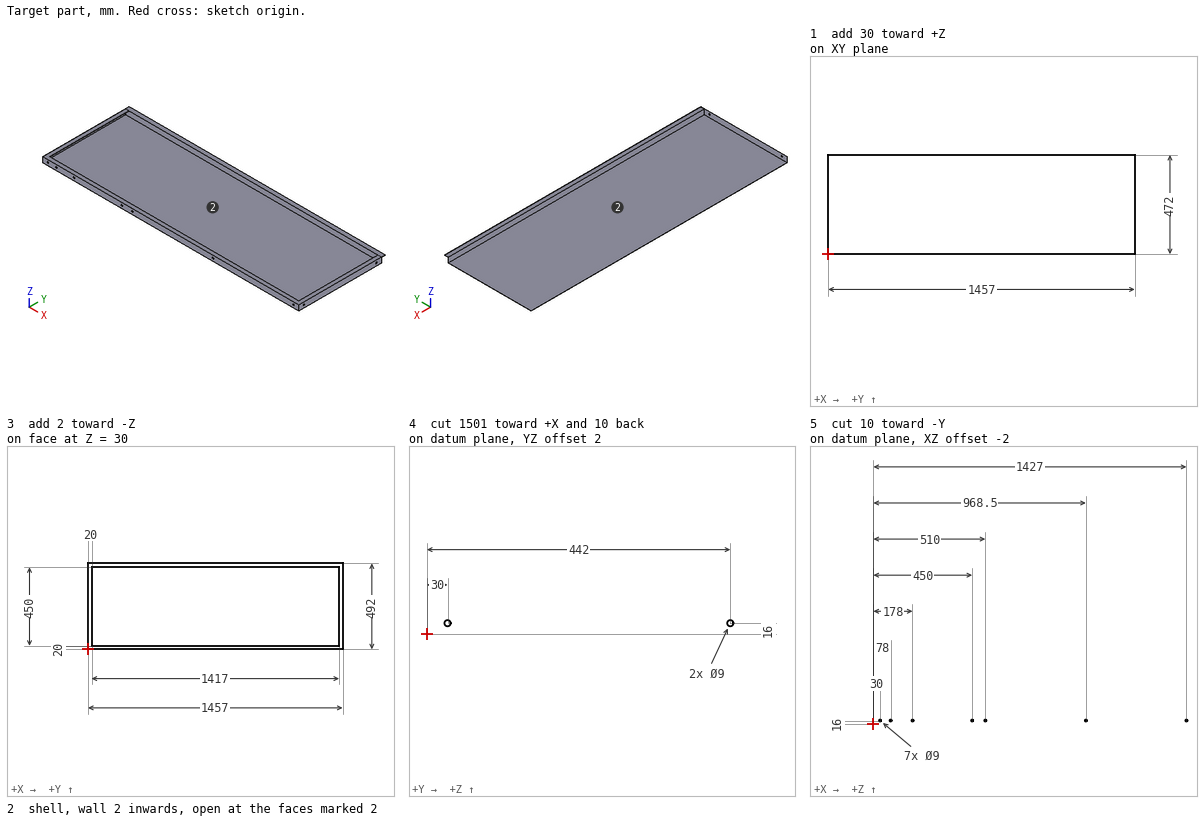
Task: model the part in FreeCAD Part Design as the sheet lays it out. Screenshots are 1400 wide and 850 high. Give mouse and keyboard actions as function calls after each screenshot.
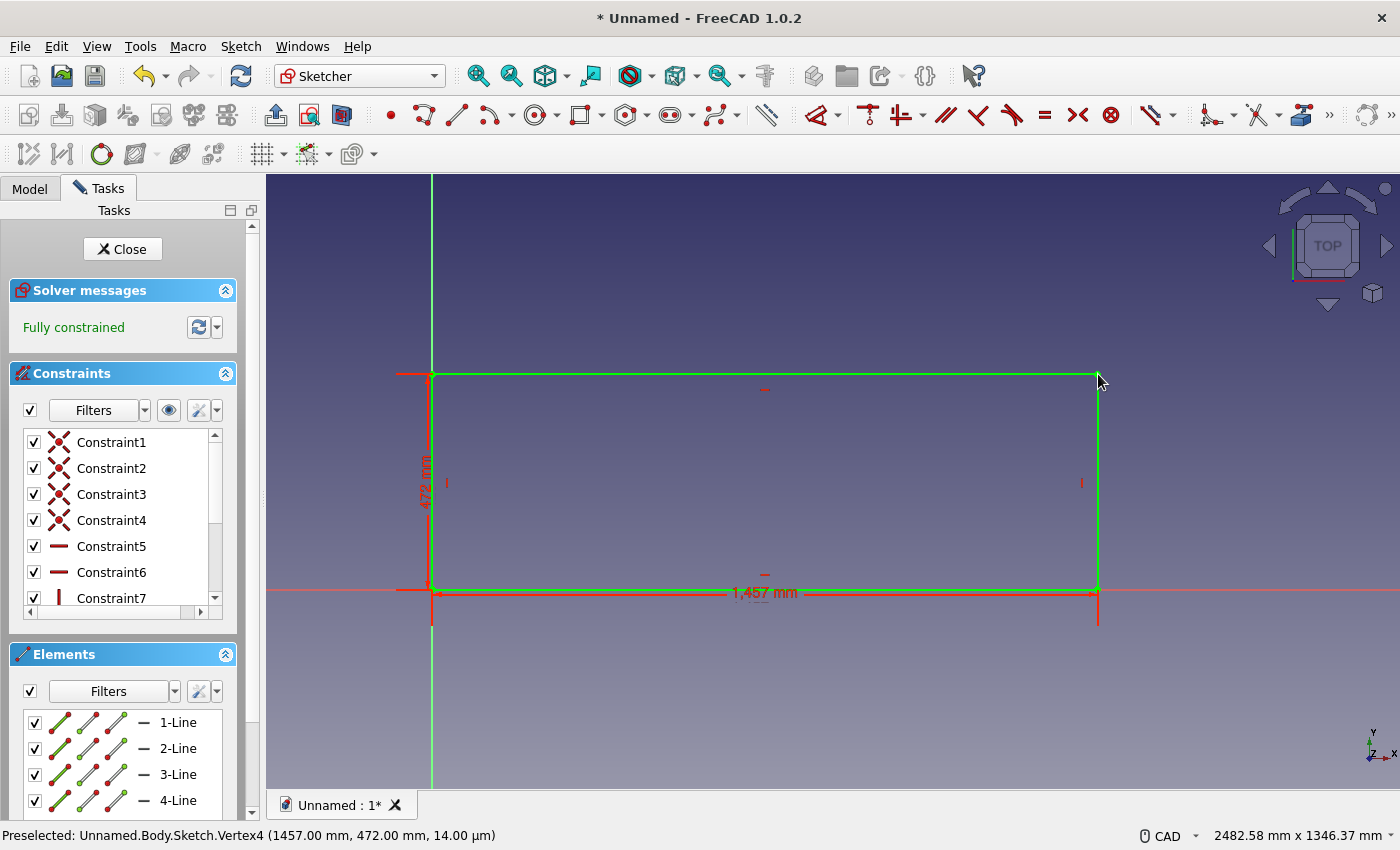
click(123, 249)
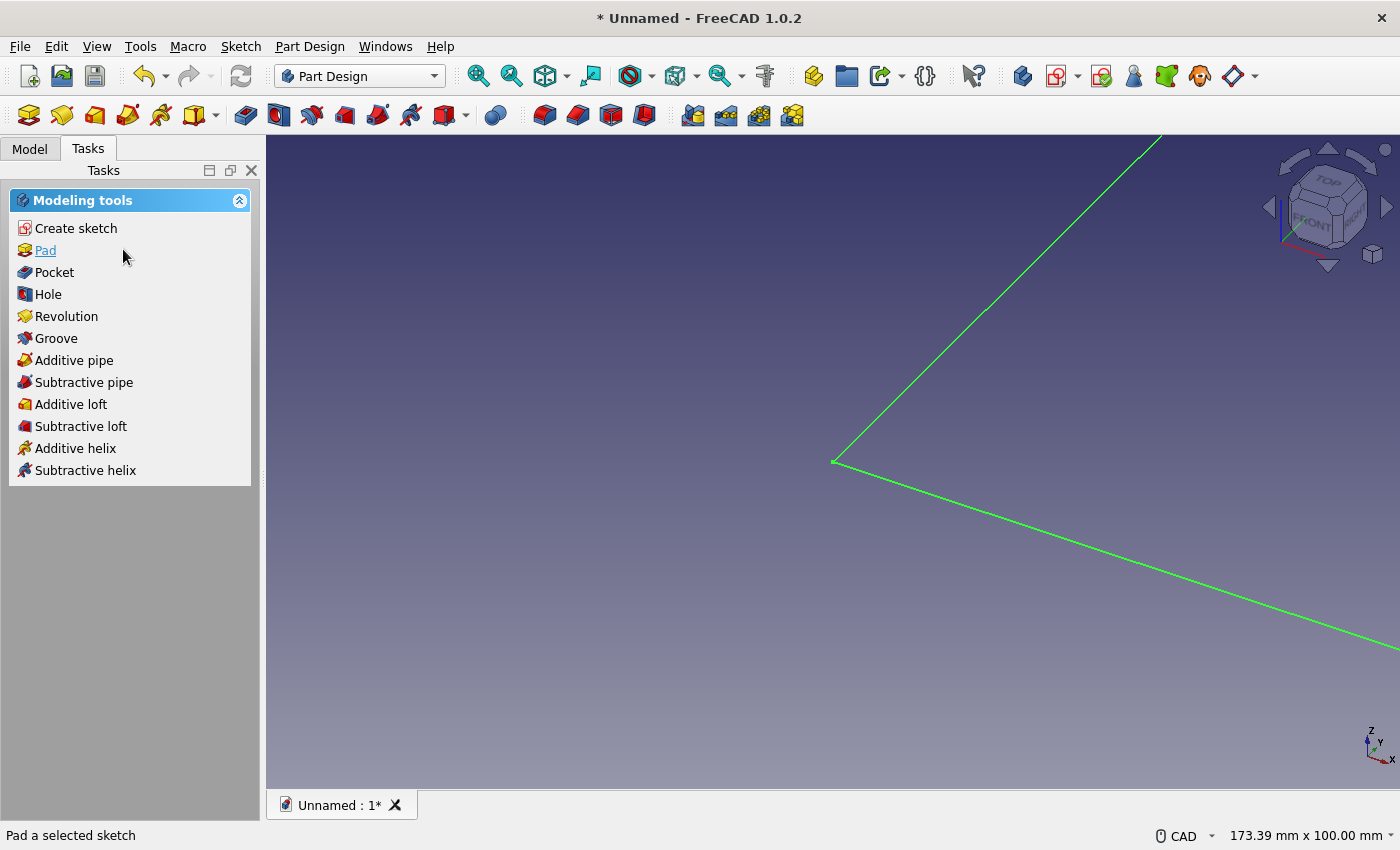
click(29, 116)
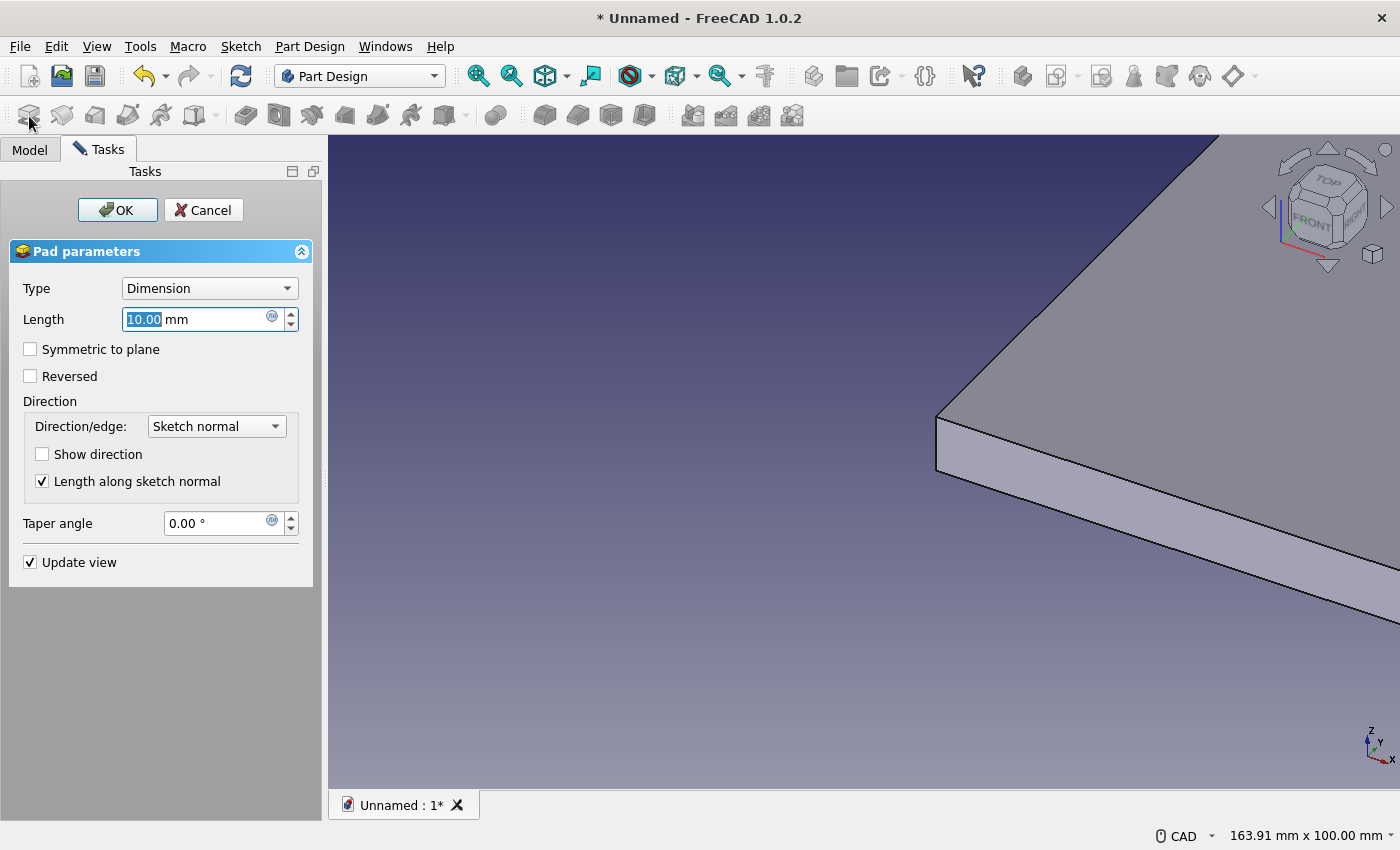
text(30)
key(Tab)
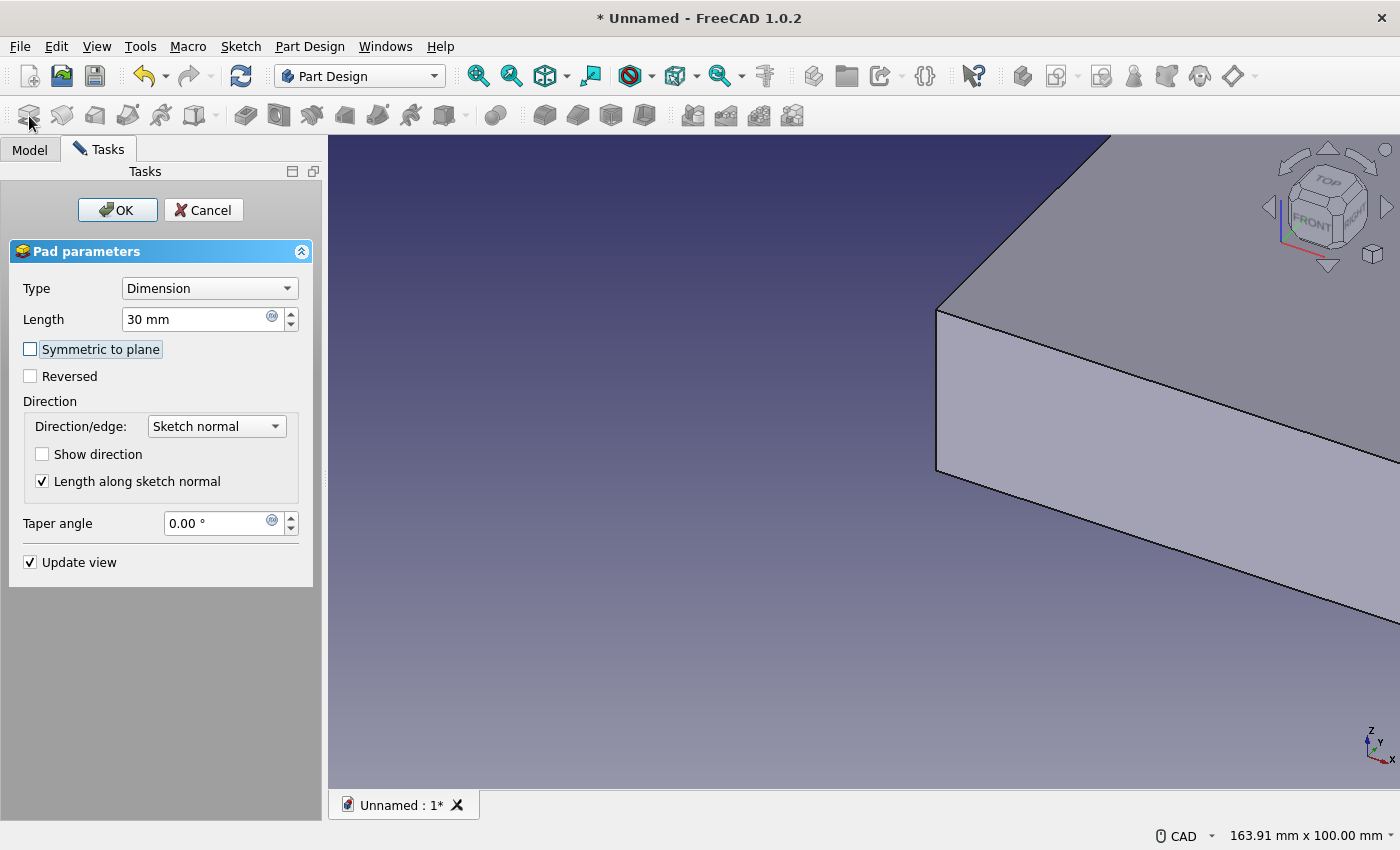
click(118, 210)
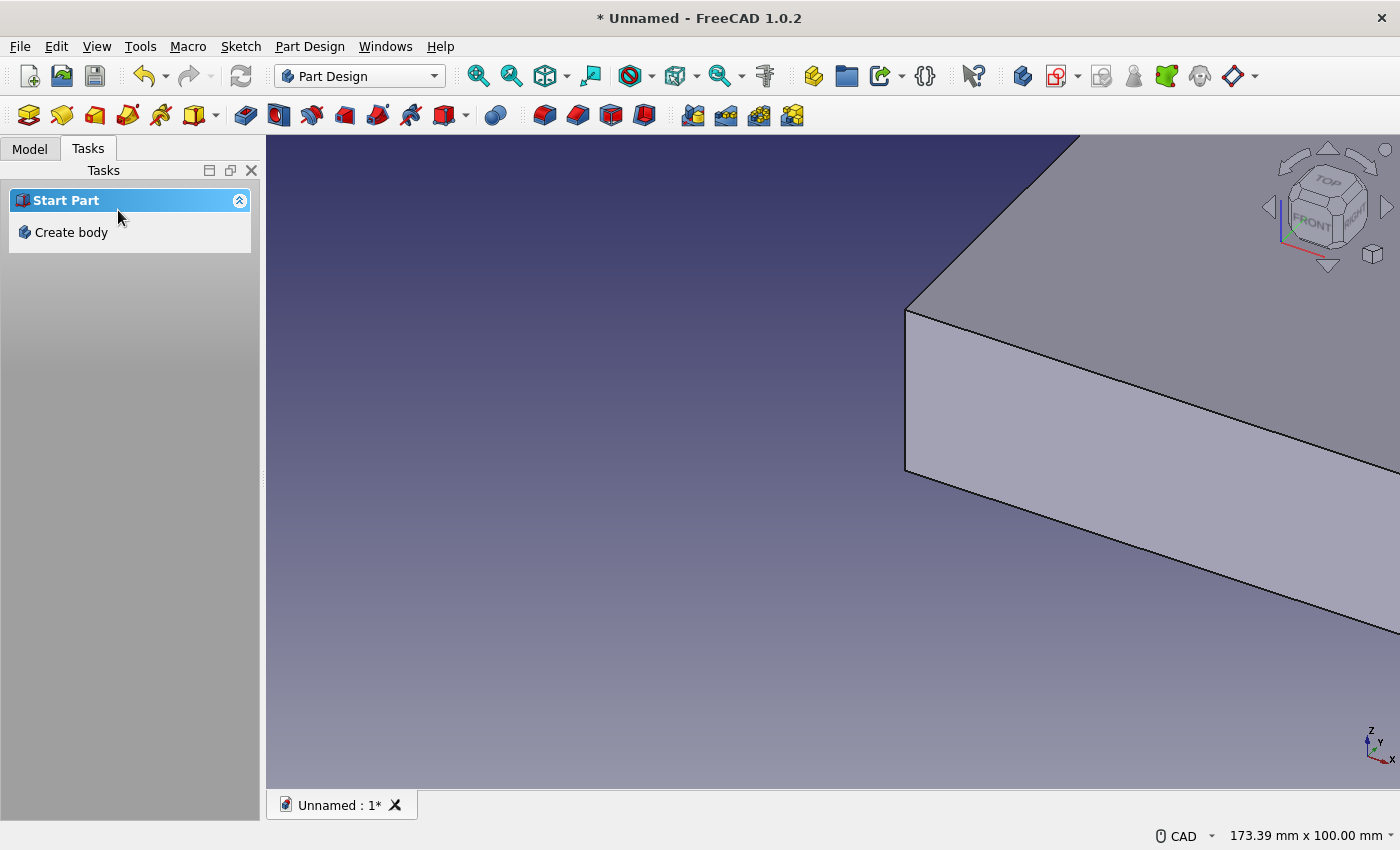
click(479, 76)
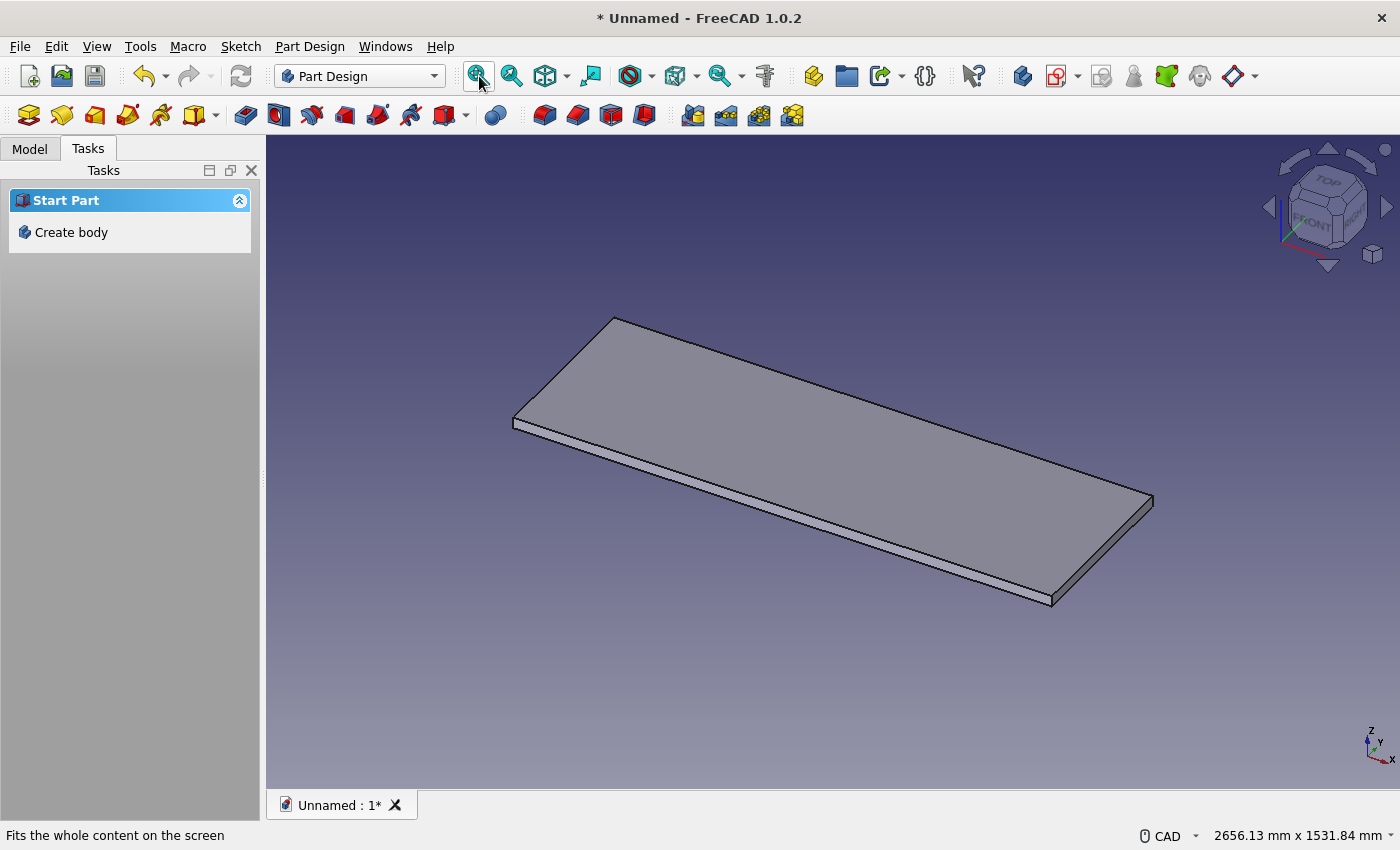
click(987, 507)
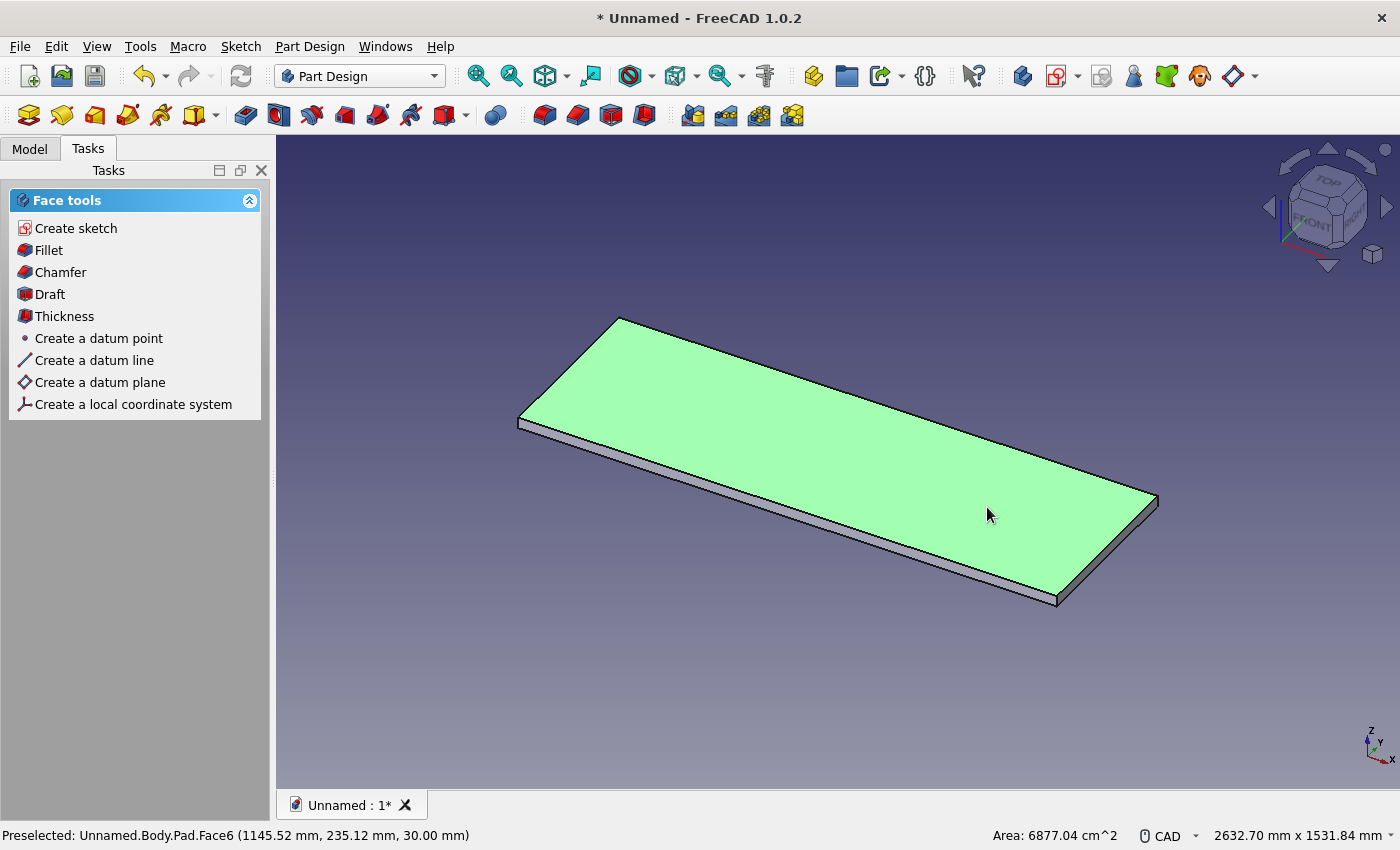
click(644, 116)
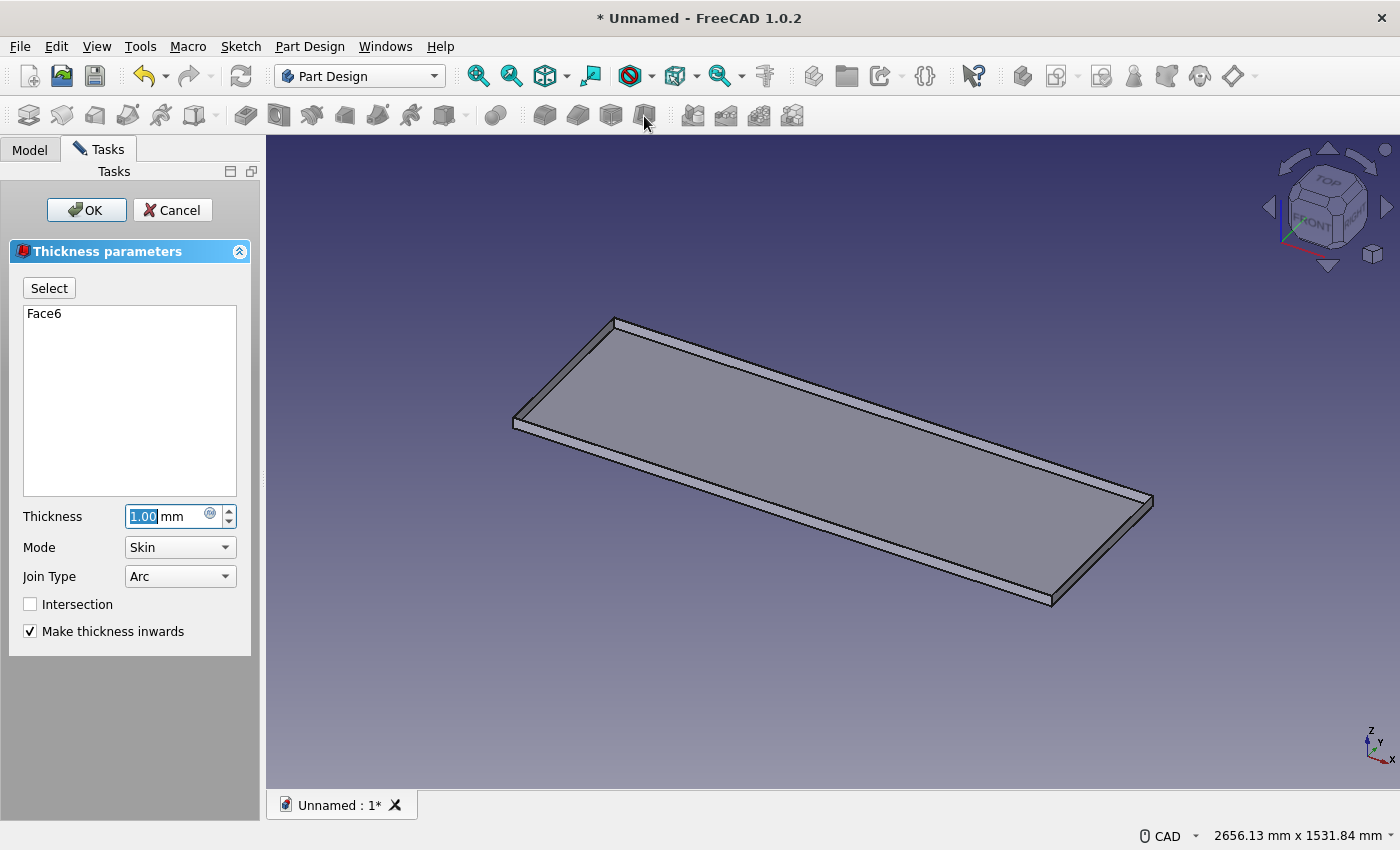
text(2)
key(Tab)